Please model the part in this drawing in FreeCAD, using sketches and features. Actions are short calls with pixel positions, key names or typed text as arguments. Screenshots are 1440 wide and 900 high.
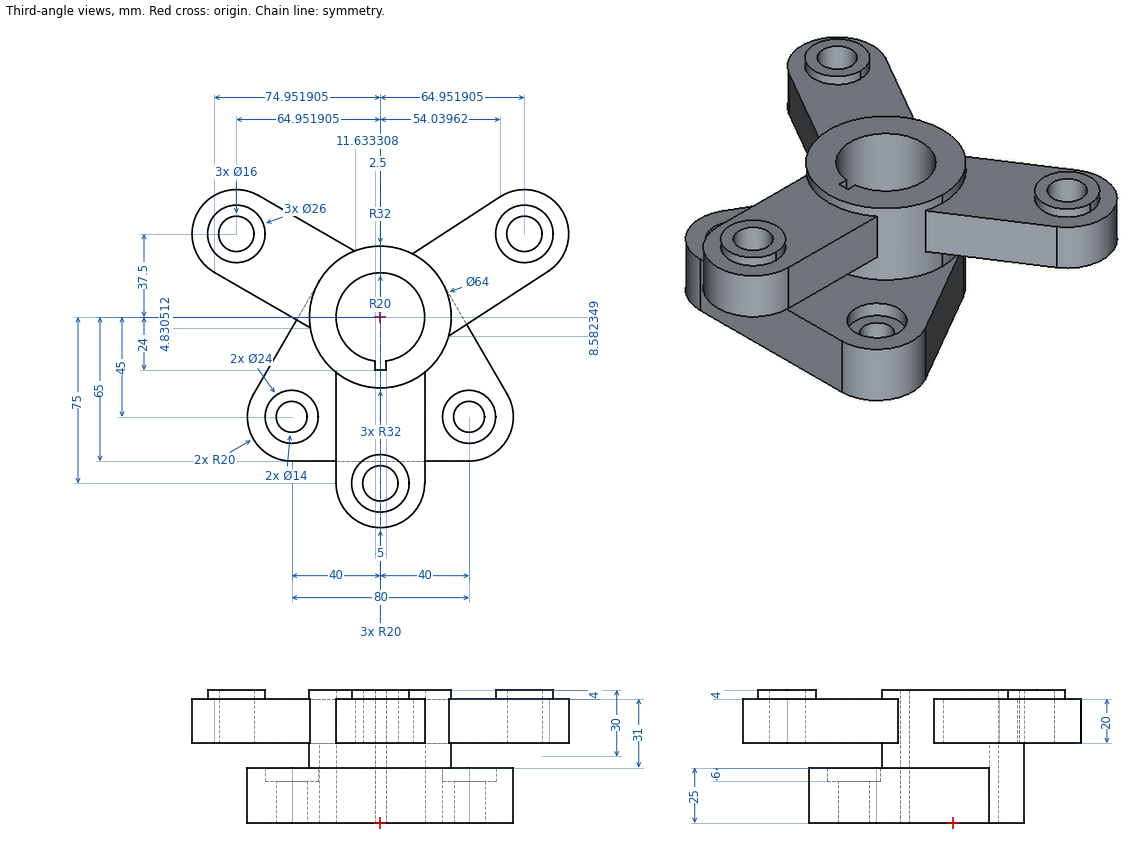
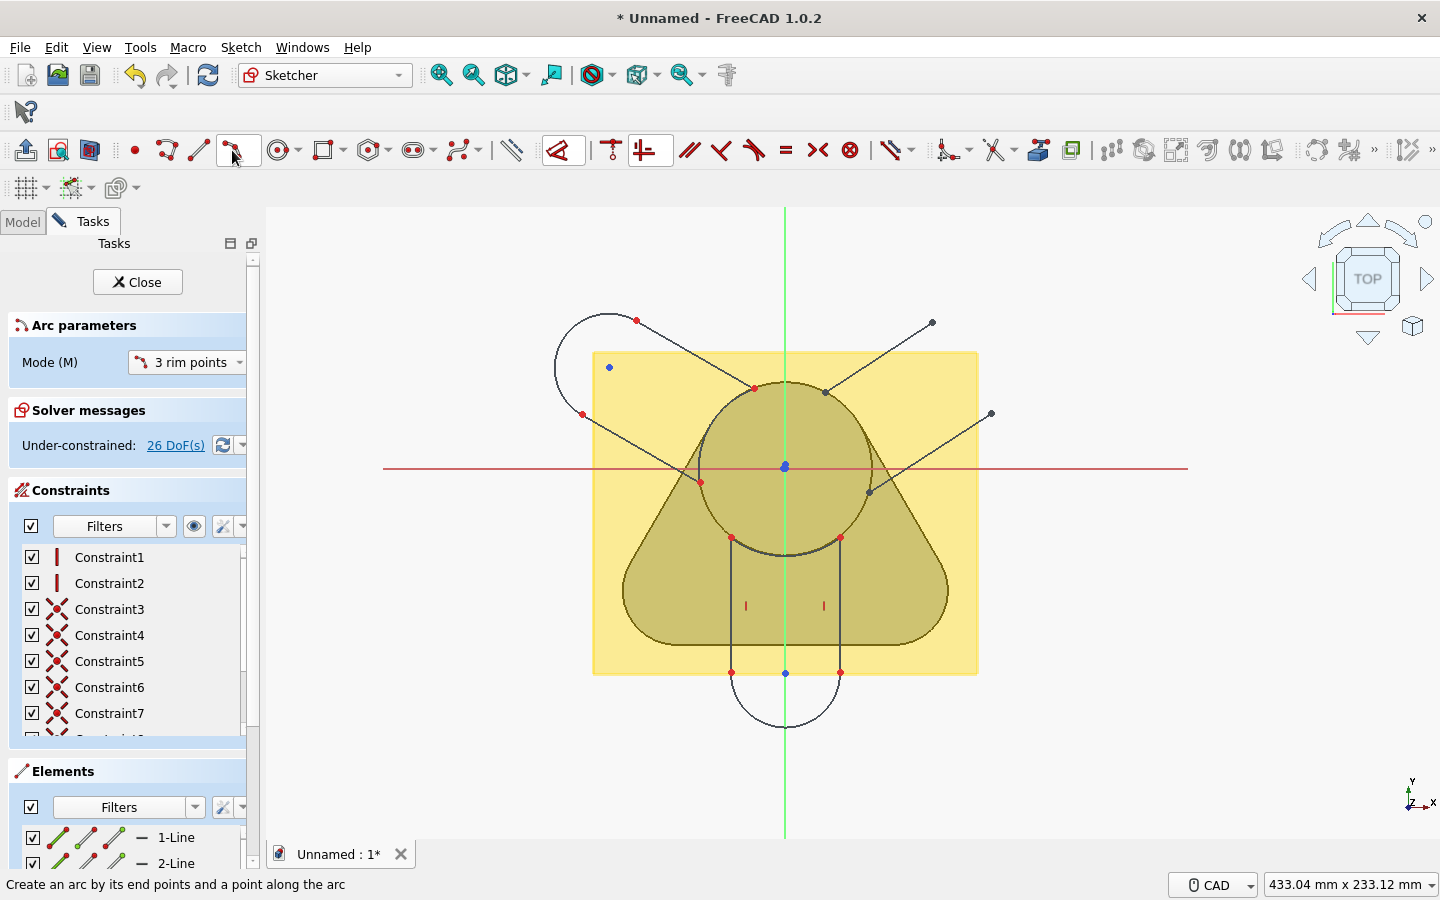
click(825, 393)
click(869, 493)
click(865, 434)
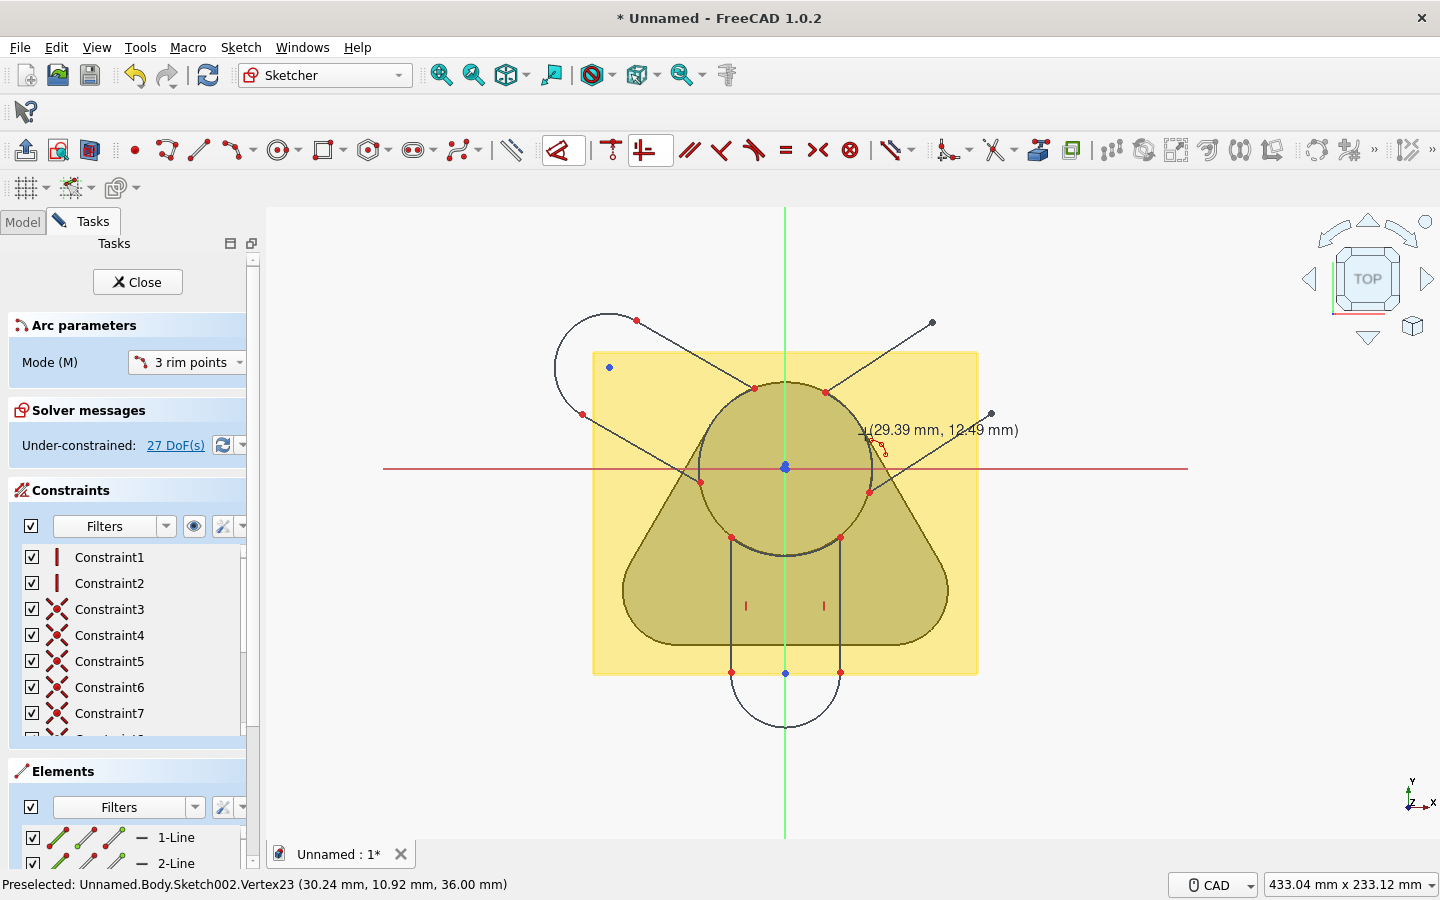
click(991, 414)
click(932, 323)
click(1007, 338)
key(Escape)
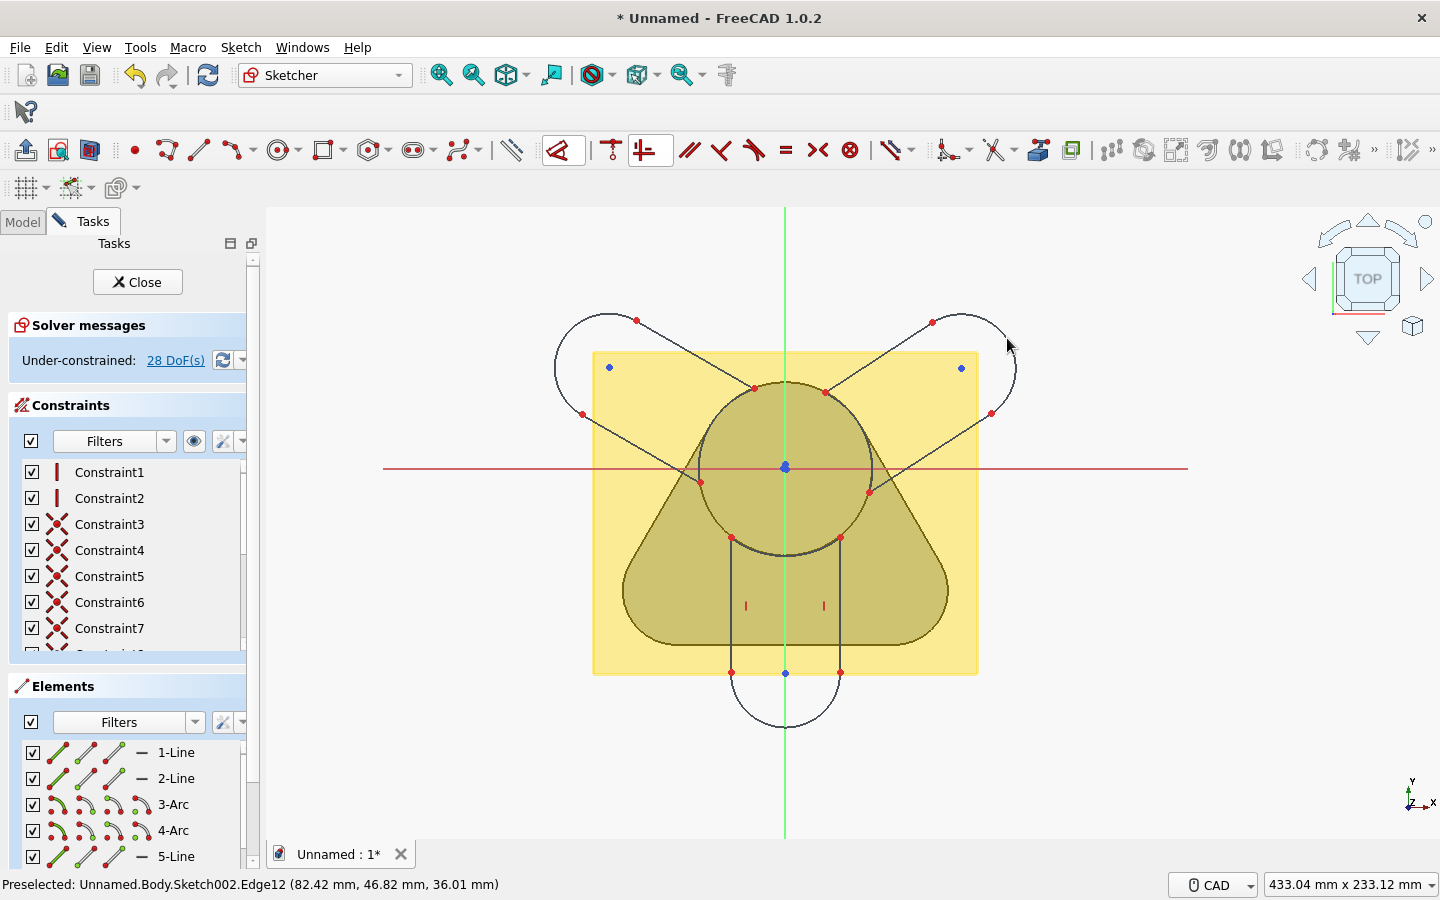
click(731, 578)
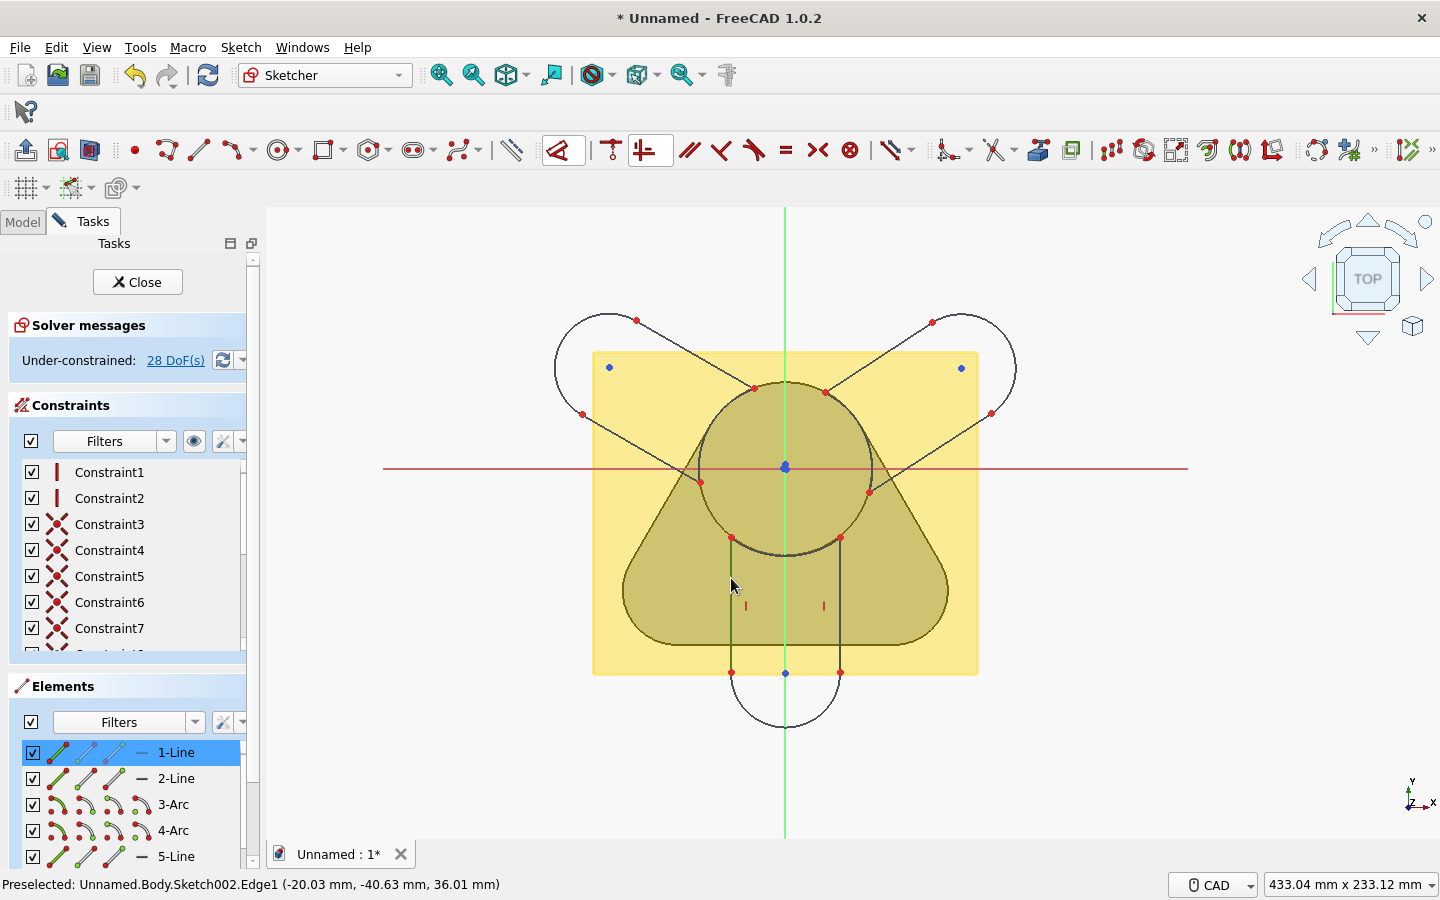
click(753, 717)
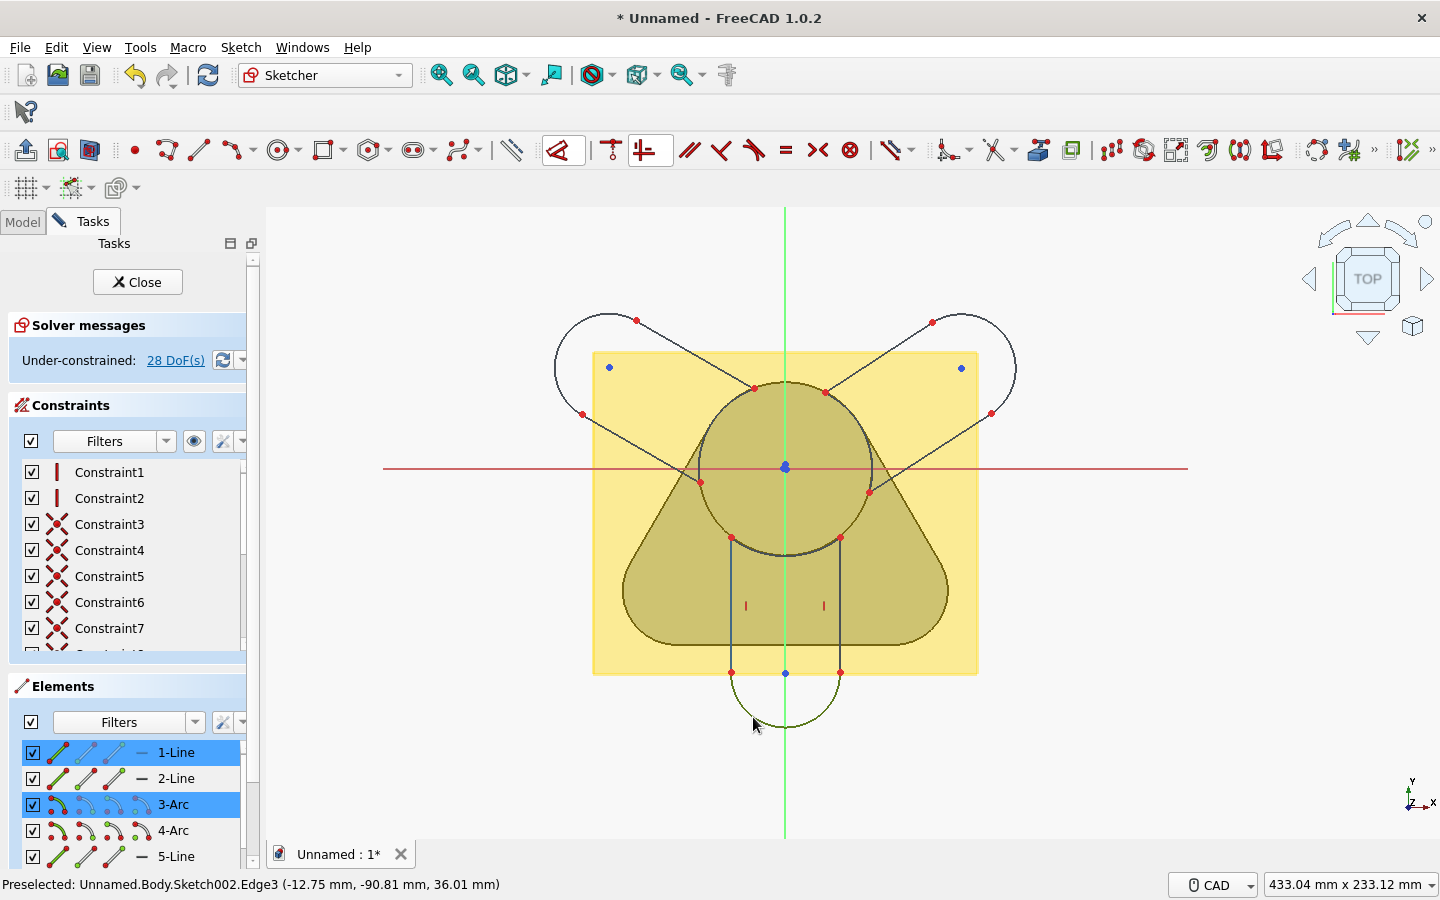
click(754, 150)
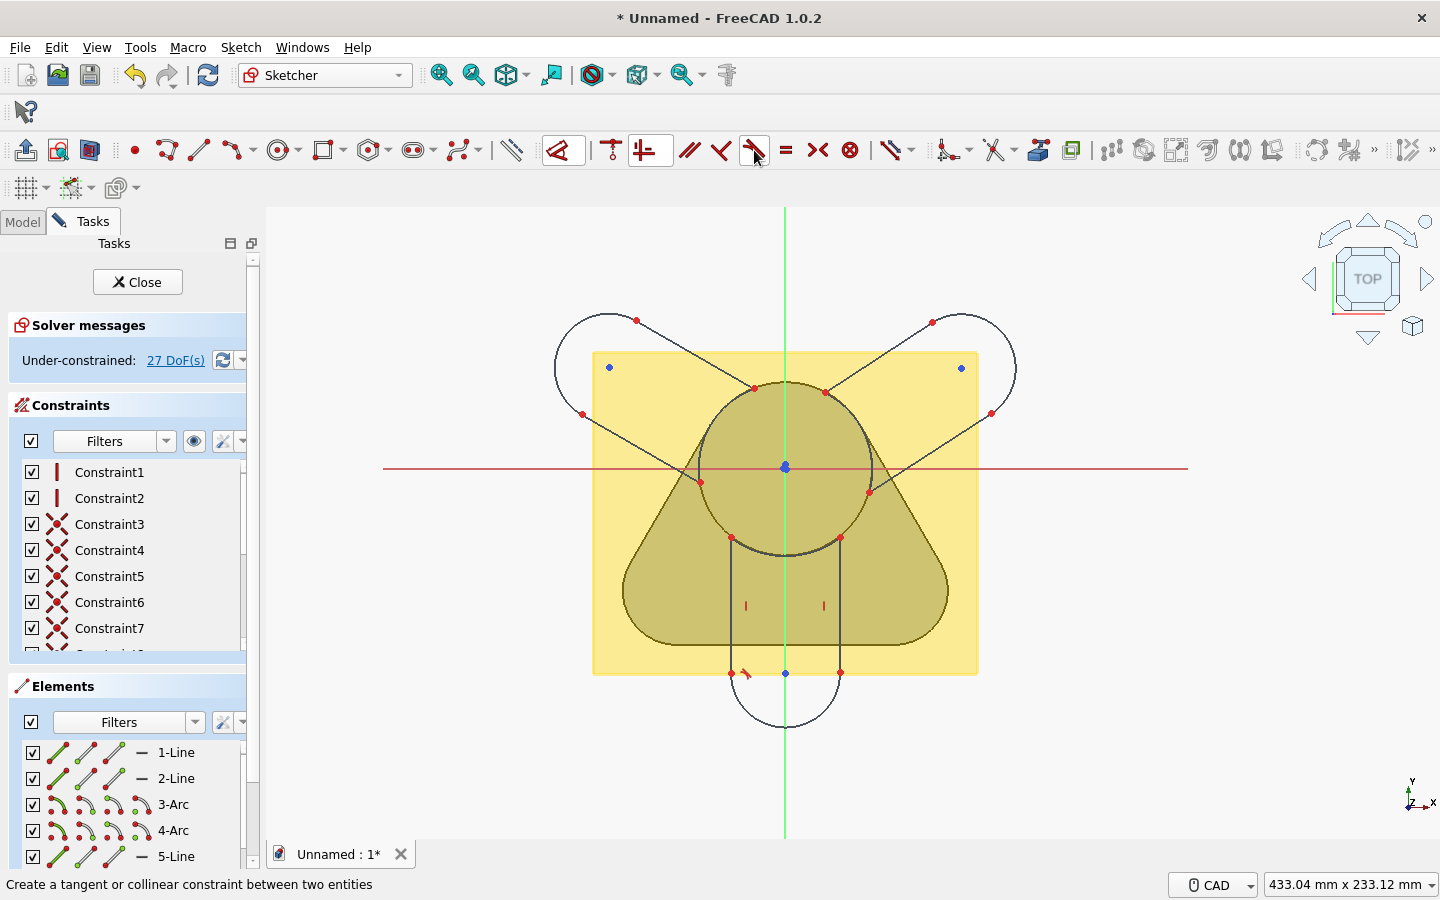
click(840, 633)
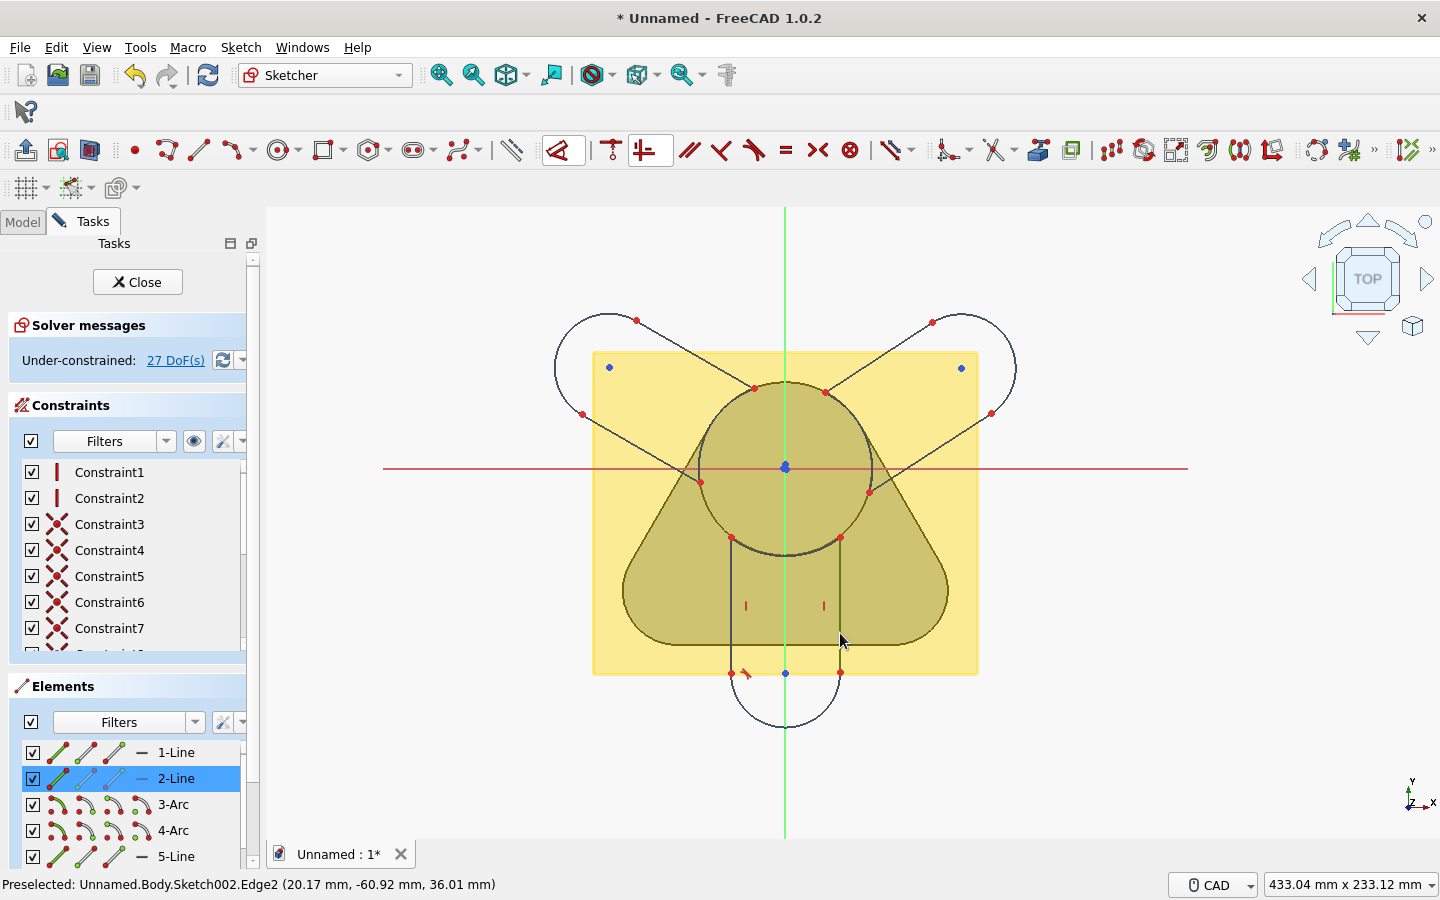
click(753, 717)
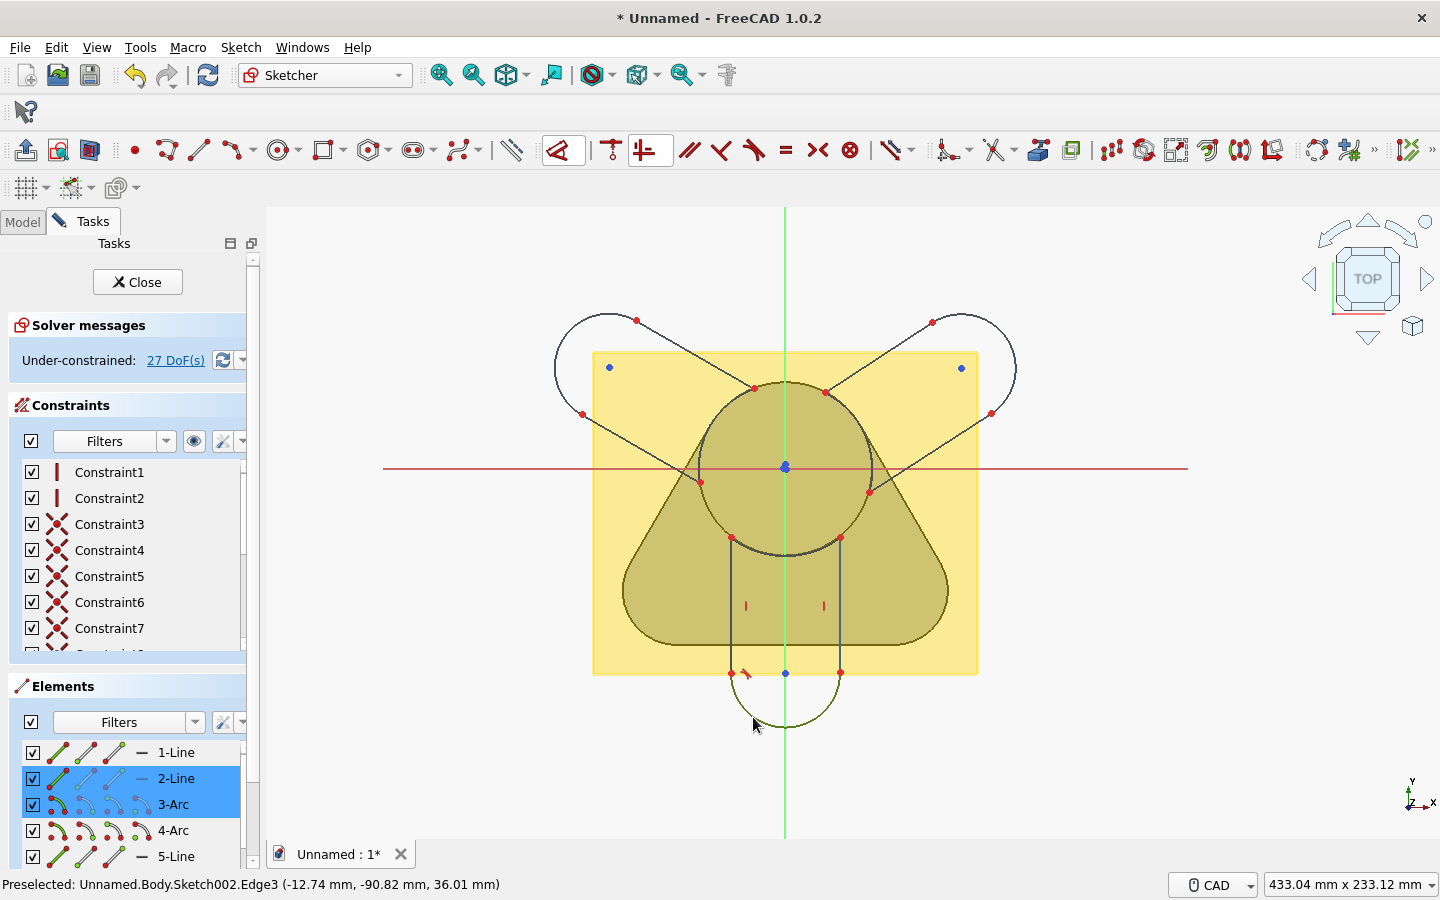
click(754, 150)